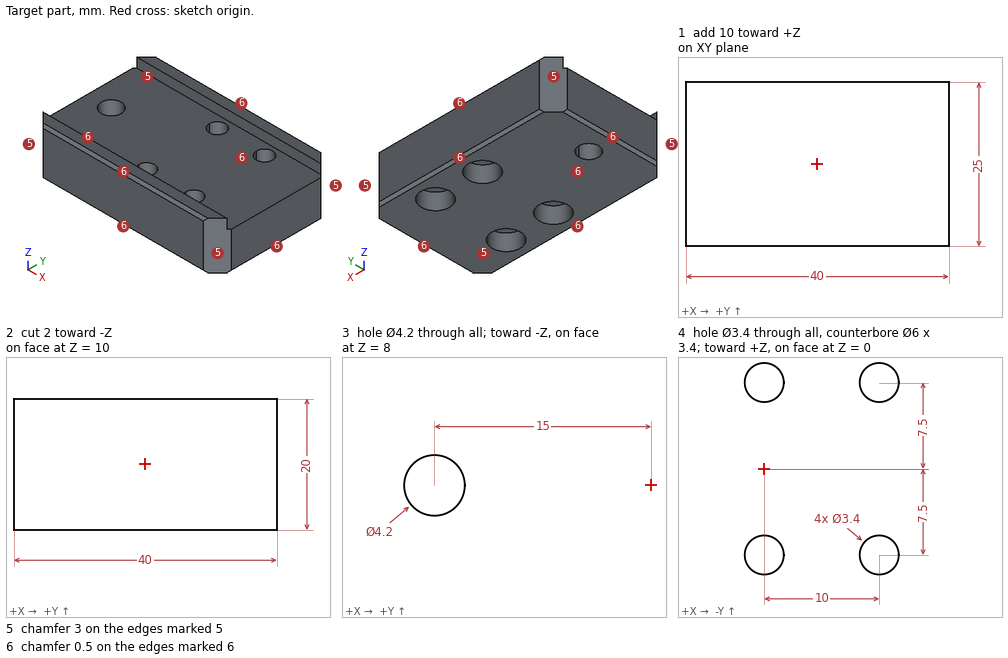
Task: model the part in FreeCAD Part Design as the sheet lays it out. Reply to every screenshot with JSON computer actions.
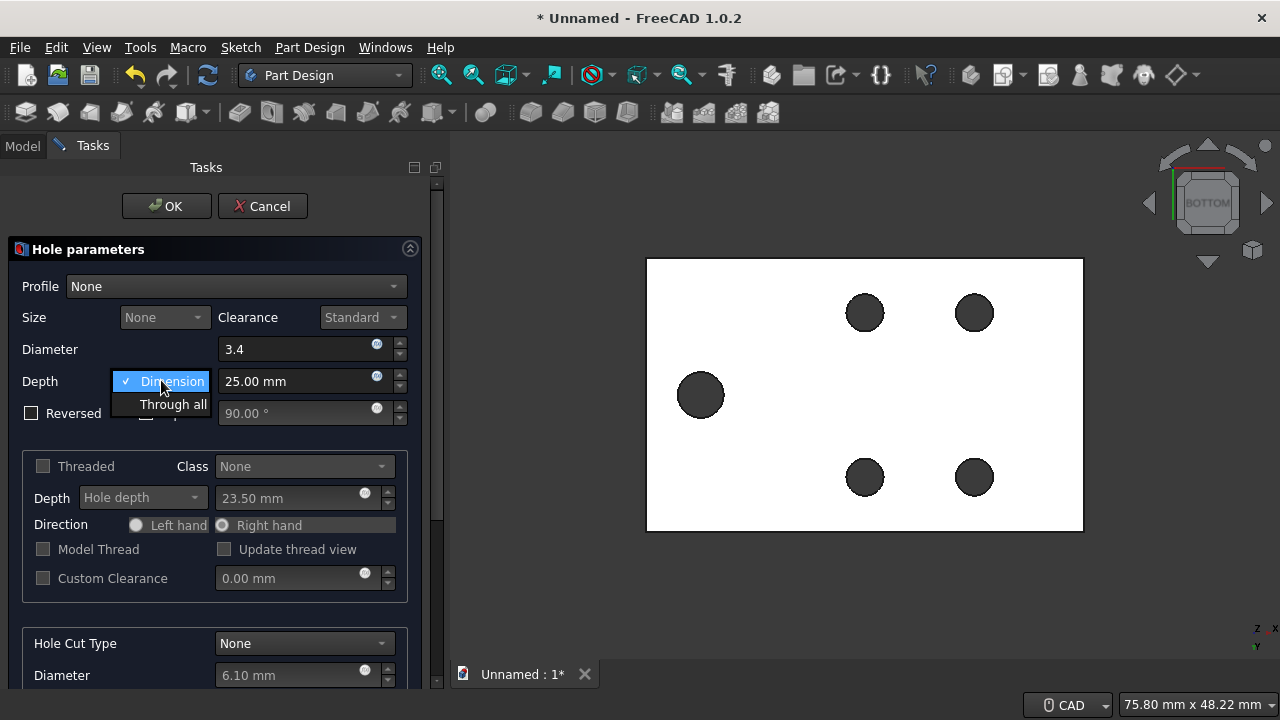
{"action": "left_click", "coordinate": [160, 404]}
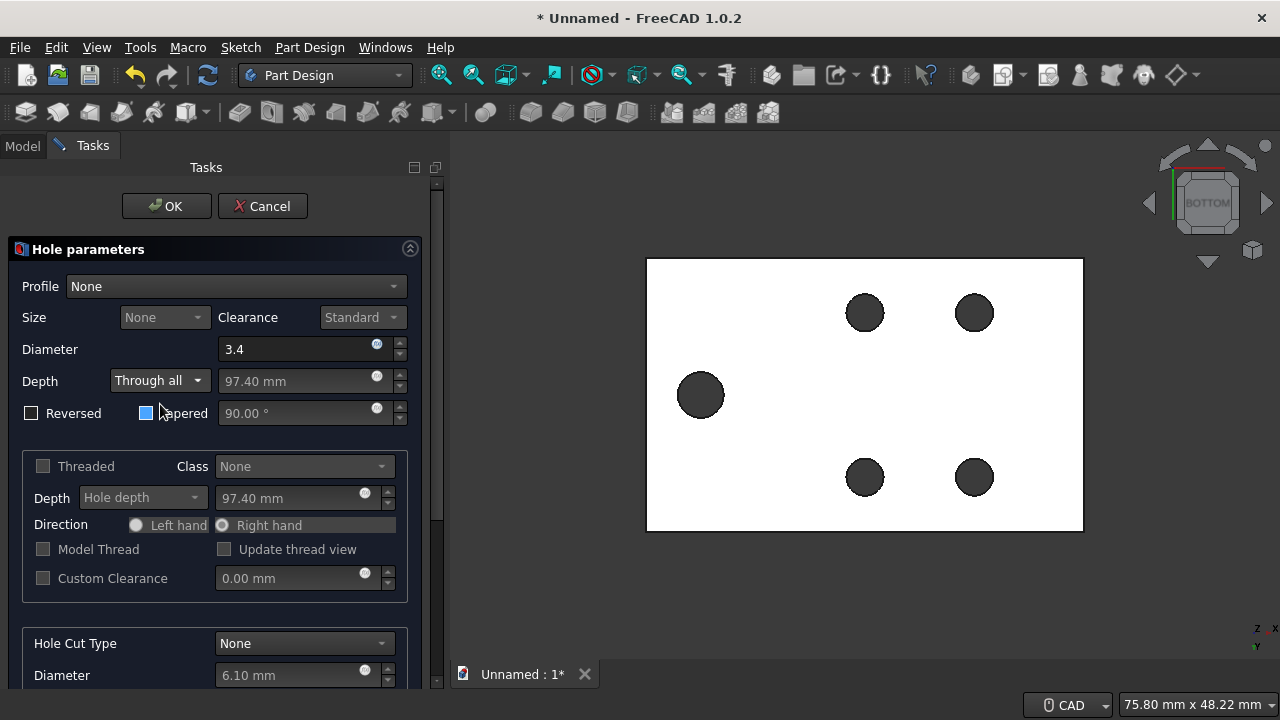
{"action": "left_click", "coordinate": [306, 644]}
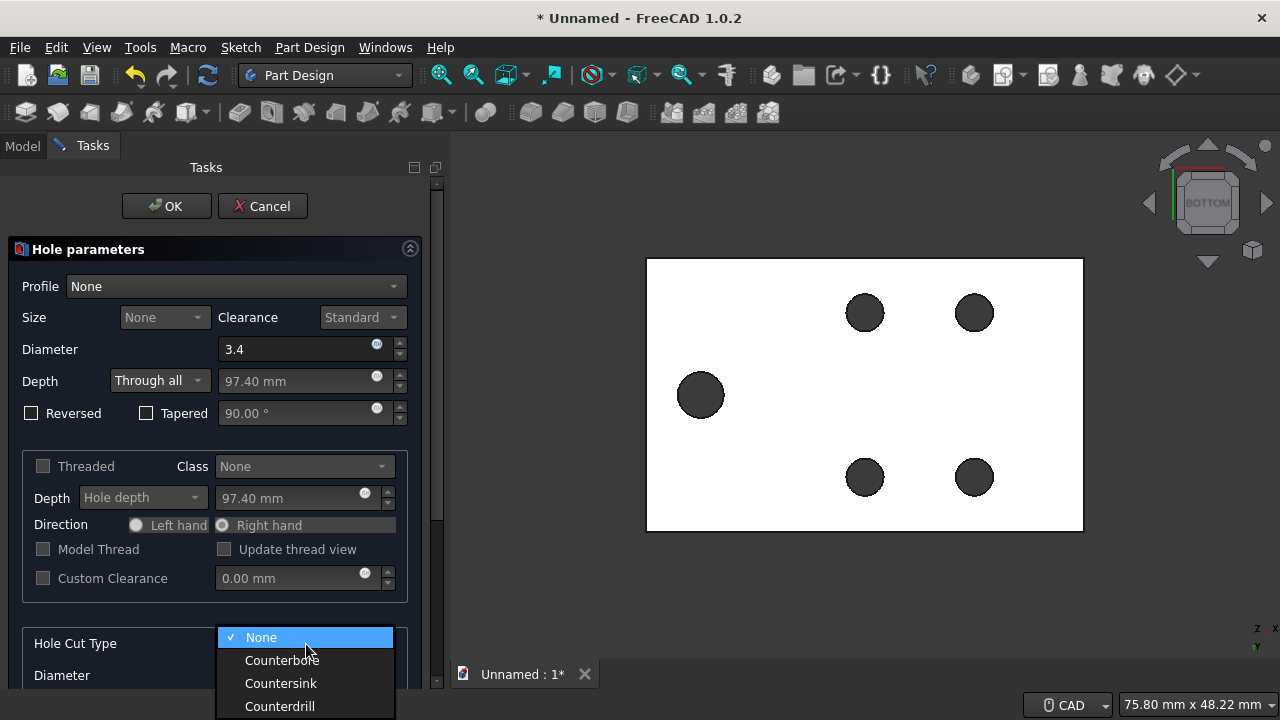
{"action": "left_click", "coordinate": [304, 660]}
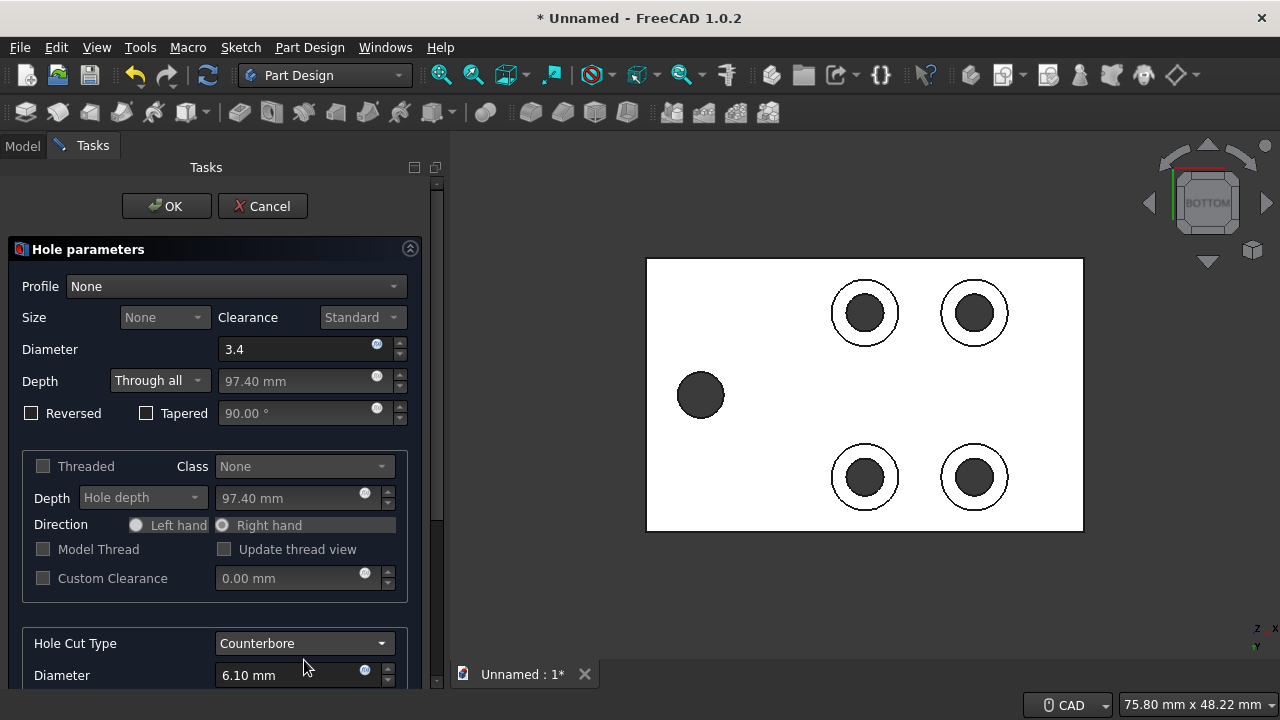
{"action": "triple_click", "coordinate": [298, 675]}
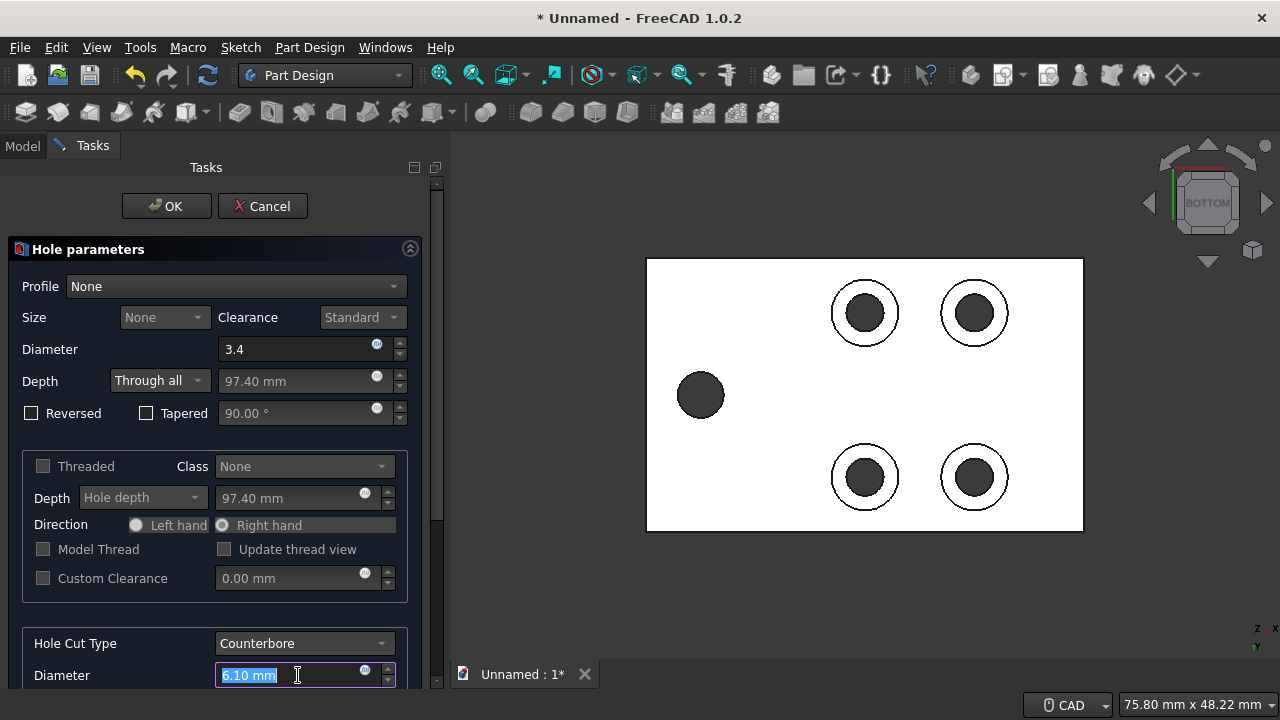
{"action": "type", "text": "6"}
{"action": "key", "text": "Tab"}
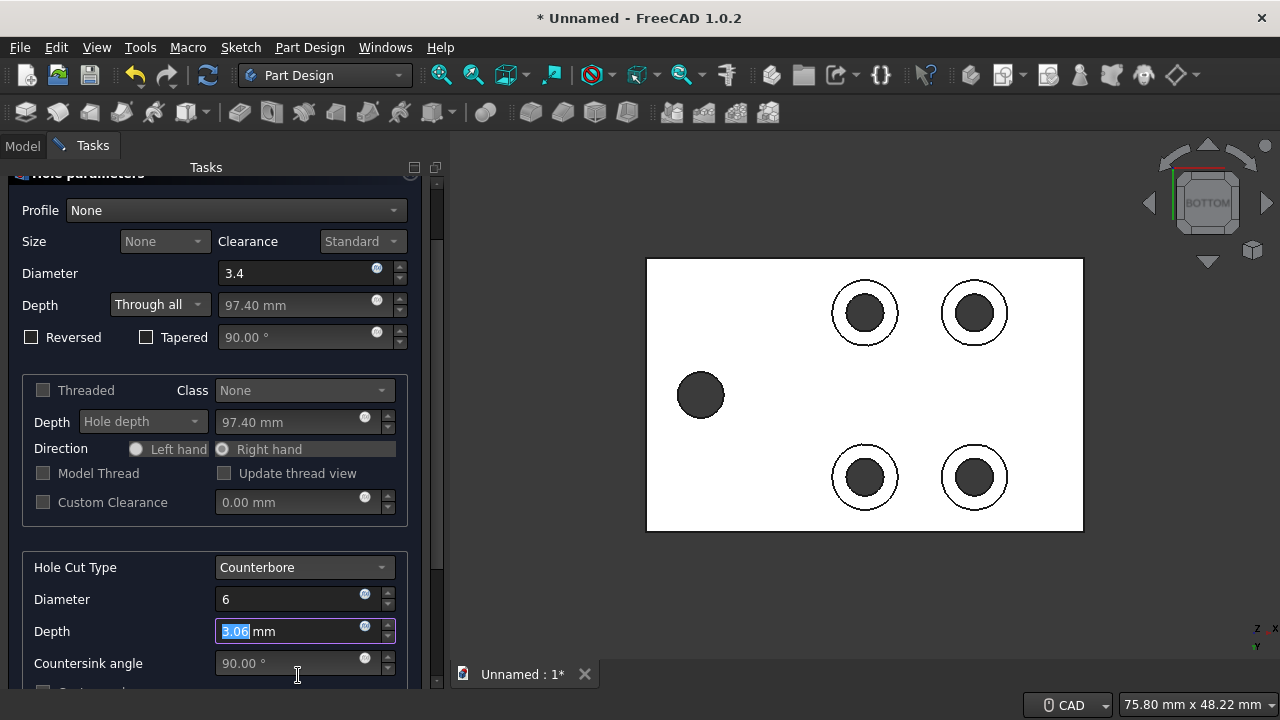
{"action": "type", "text": "3.4"}
{"action": "key", "text": "Tab"}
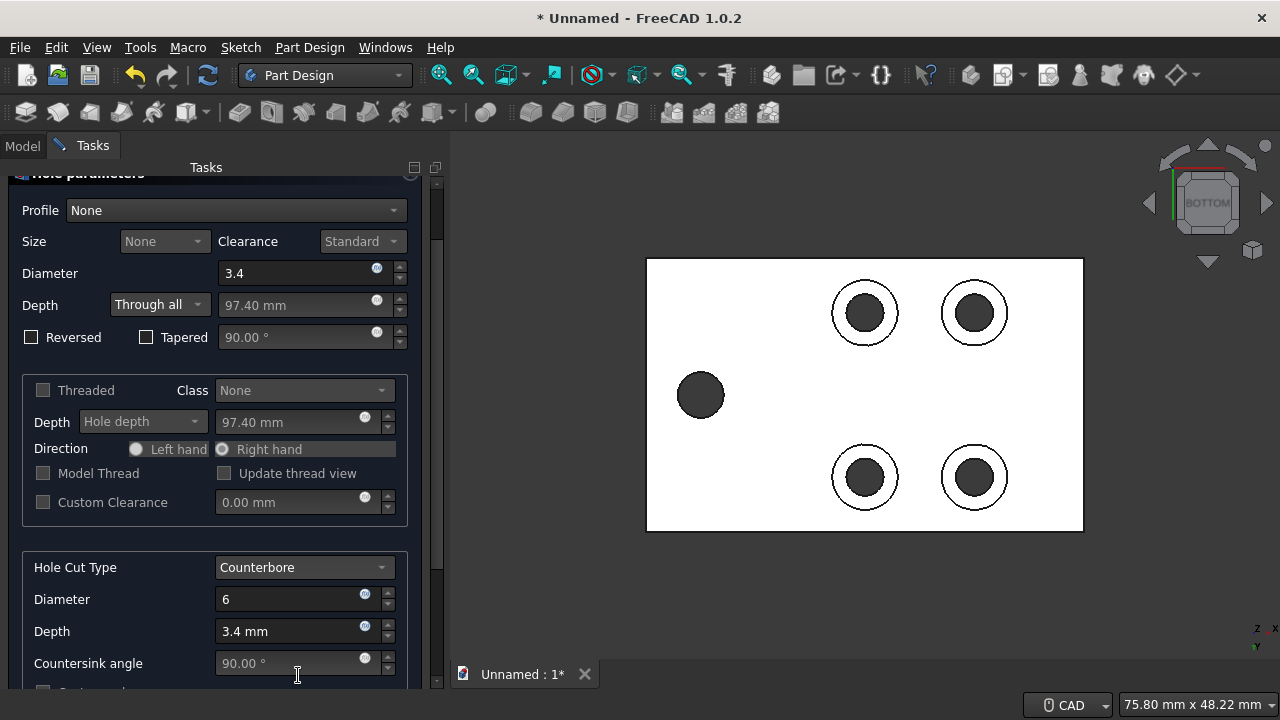
{"action": "scroll", "coordinate": [437, 432], "scroll_direction": "up", "scroll_amount": 3}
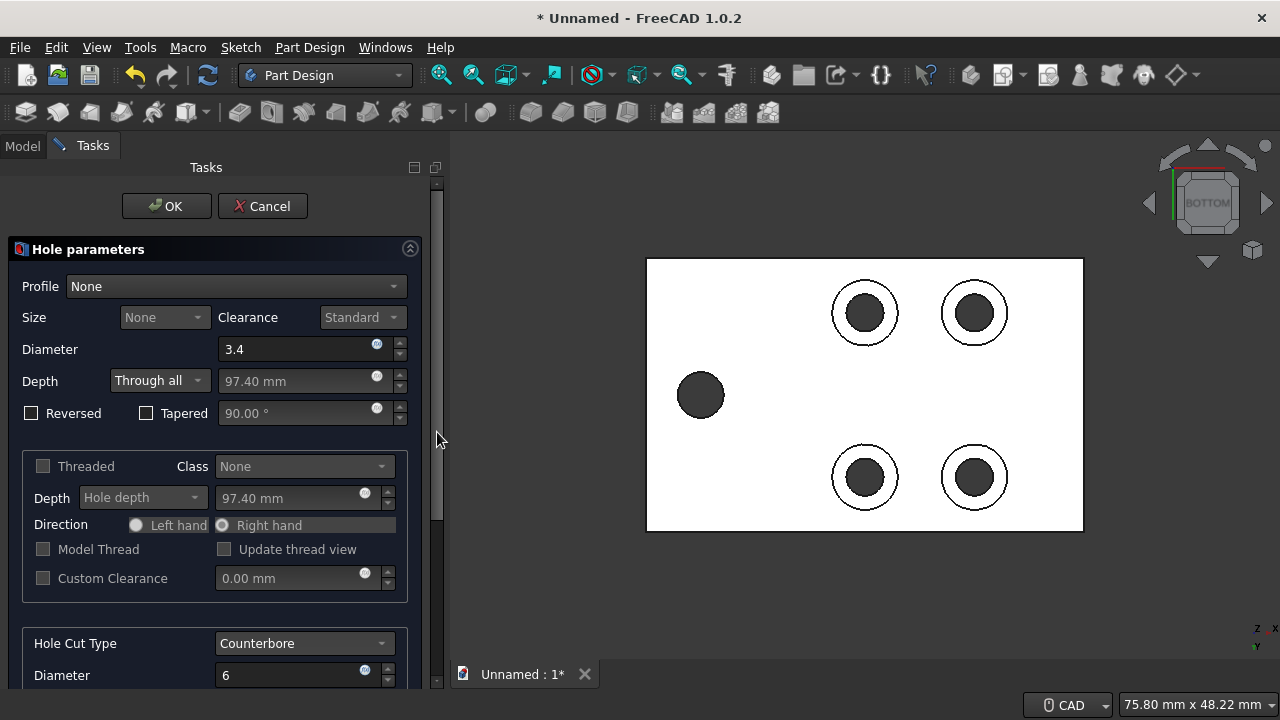
{"action": "left_click", "coordinate": [167, 206]}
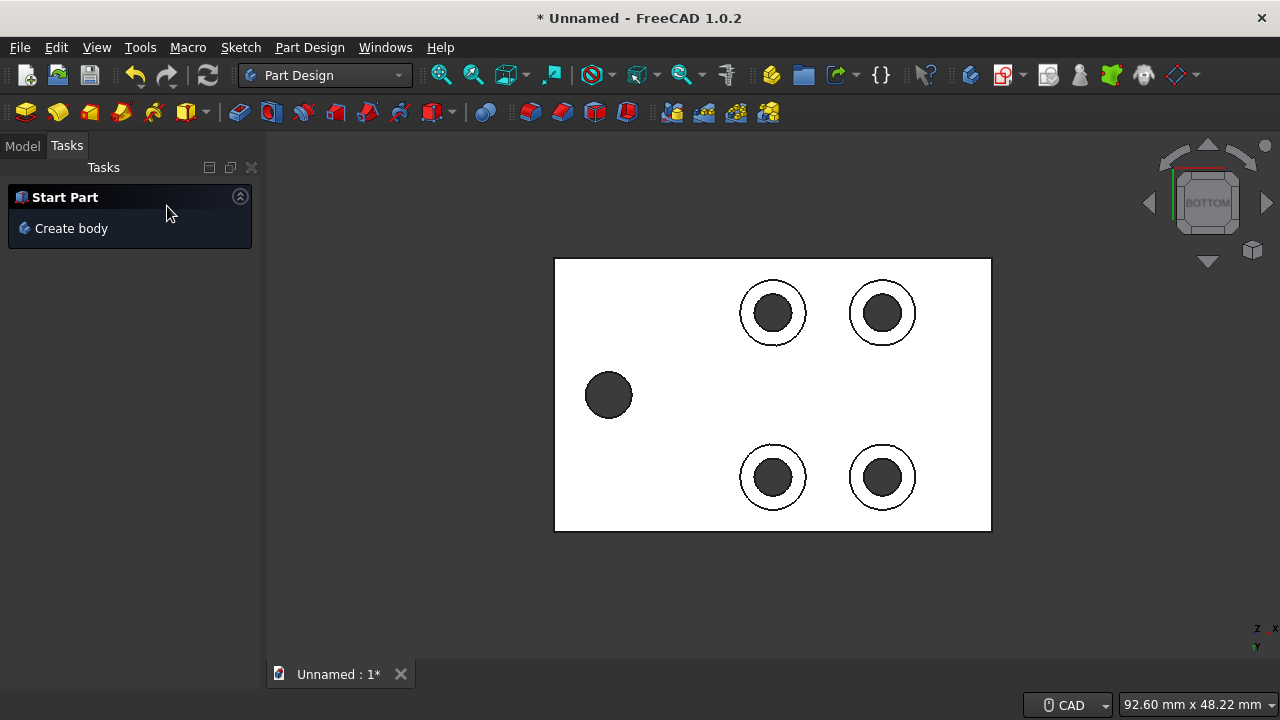
{"action": "key", "text": "0"}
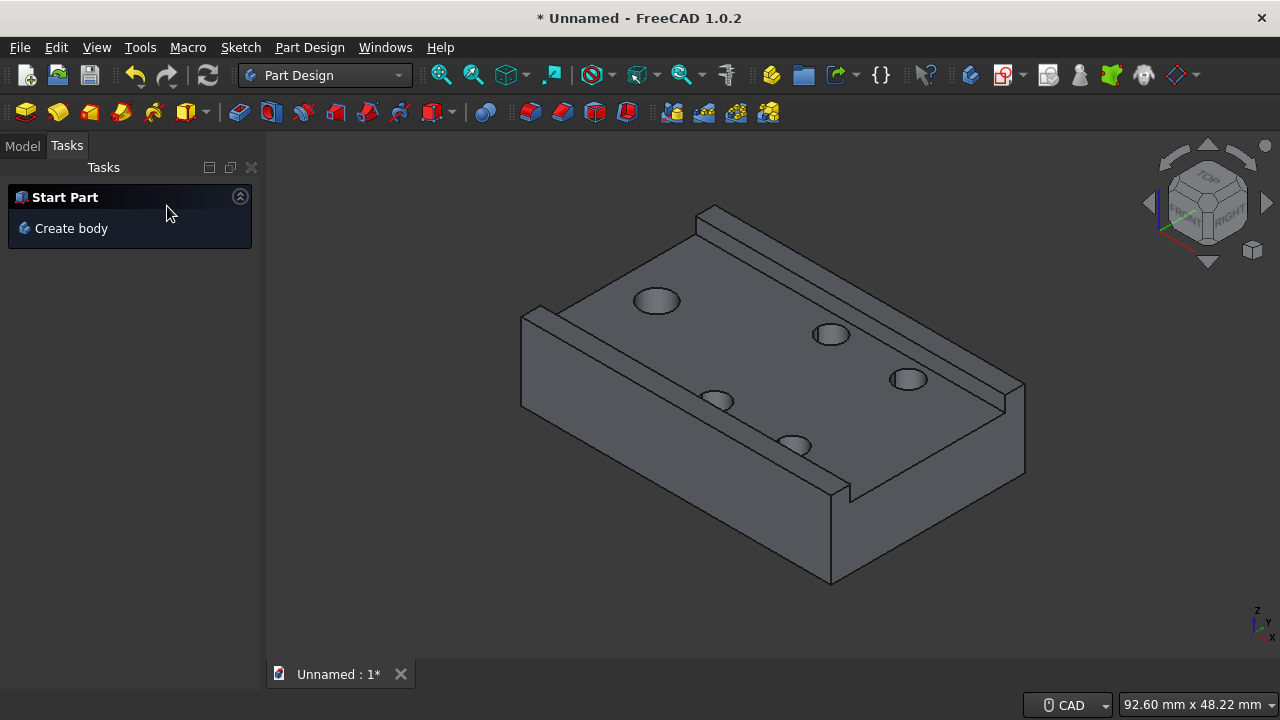
{"action": "left_click", "coordinate": [831, 539]}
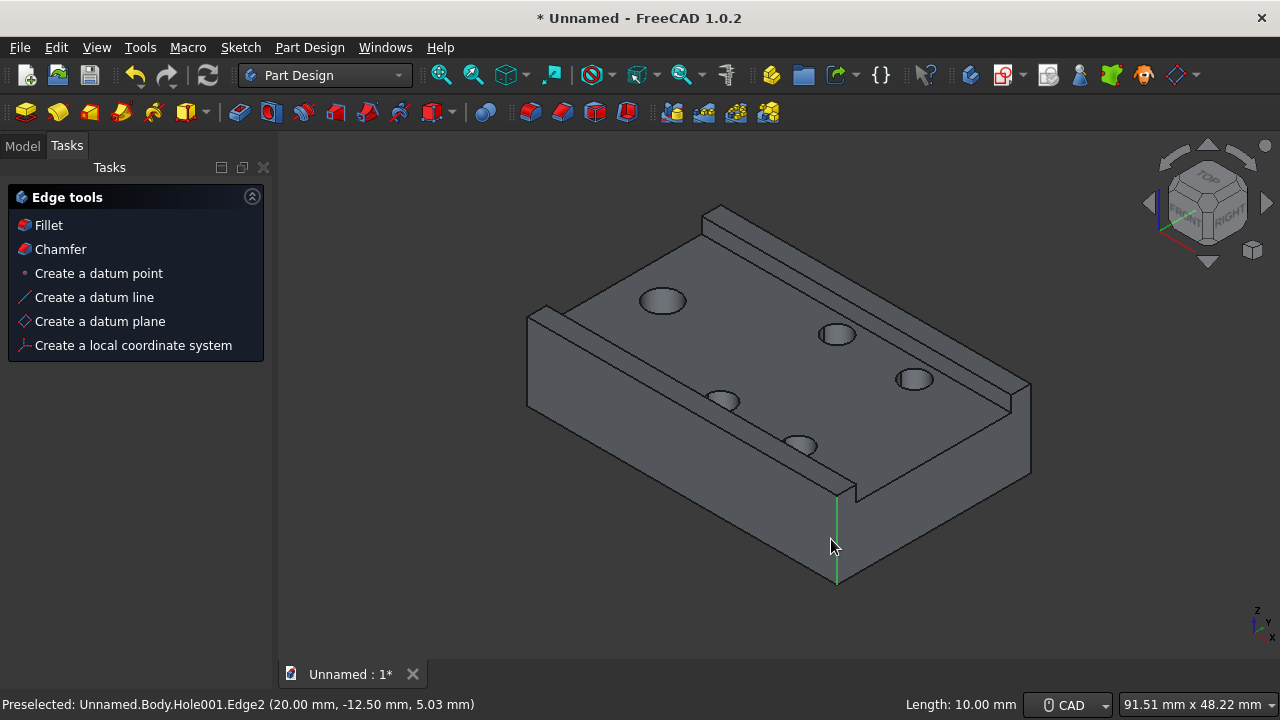
{"action": "key", "text": "2"}